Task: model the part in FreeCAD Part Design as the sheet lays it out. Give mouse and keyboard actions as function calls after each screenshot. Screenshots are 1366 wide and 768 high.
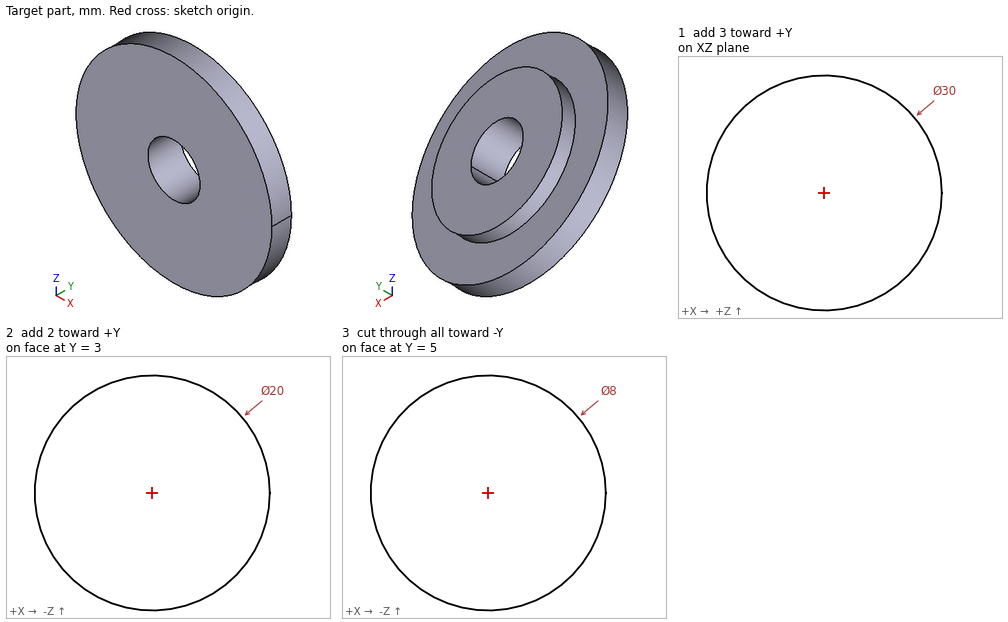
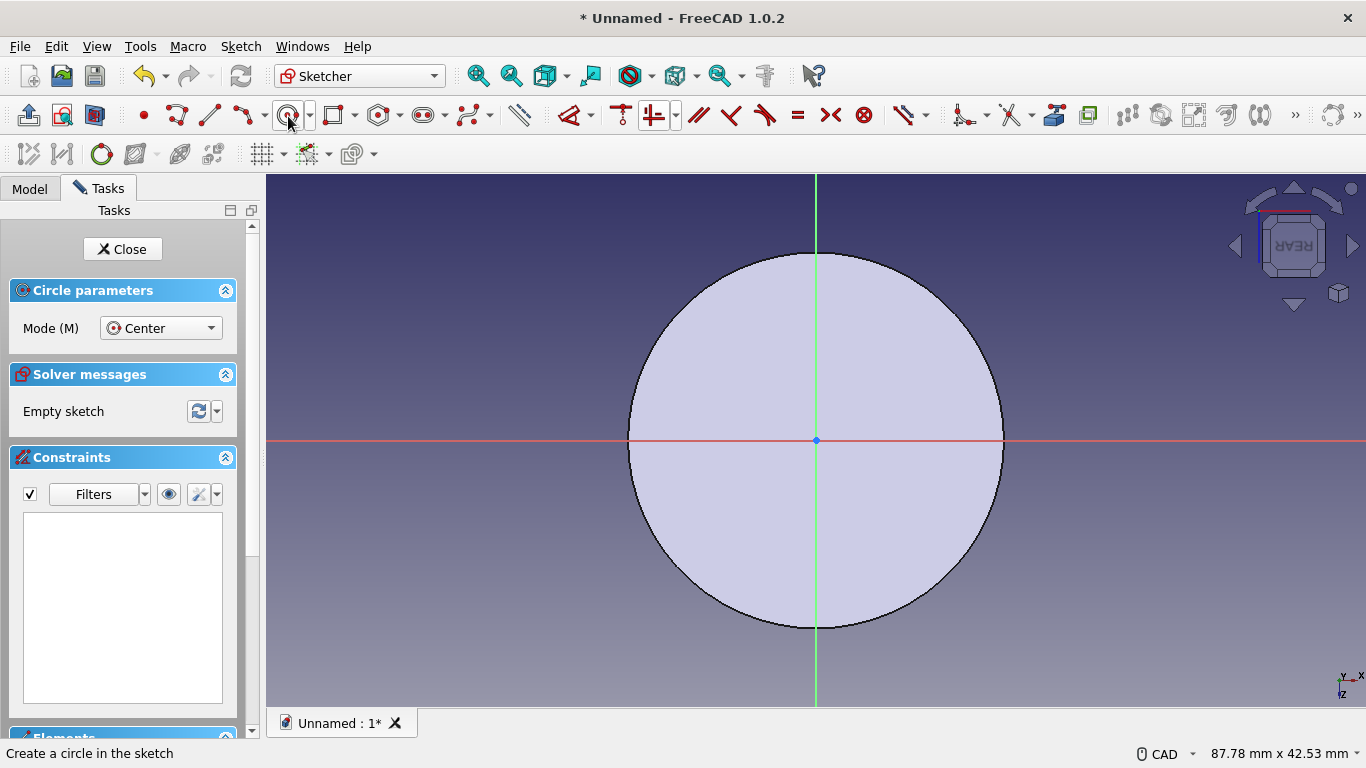
click(816, 441)
click(905, 352)
key(Escape)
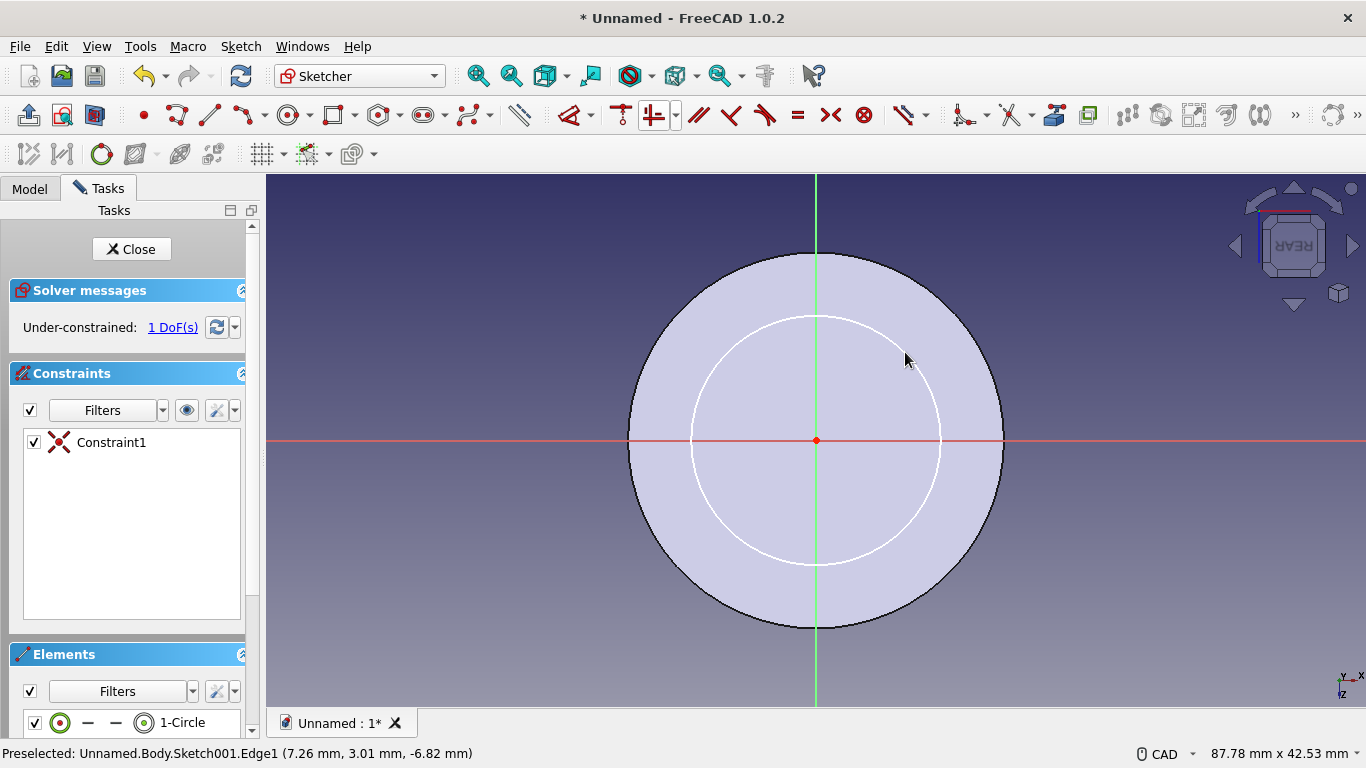
click(568, 116)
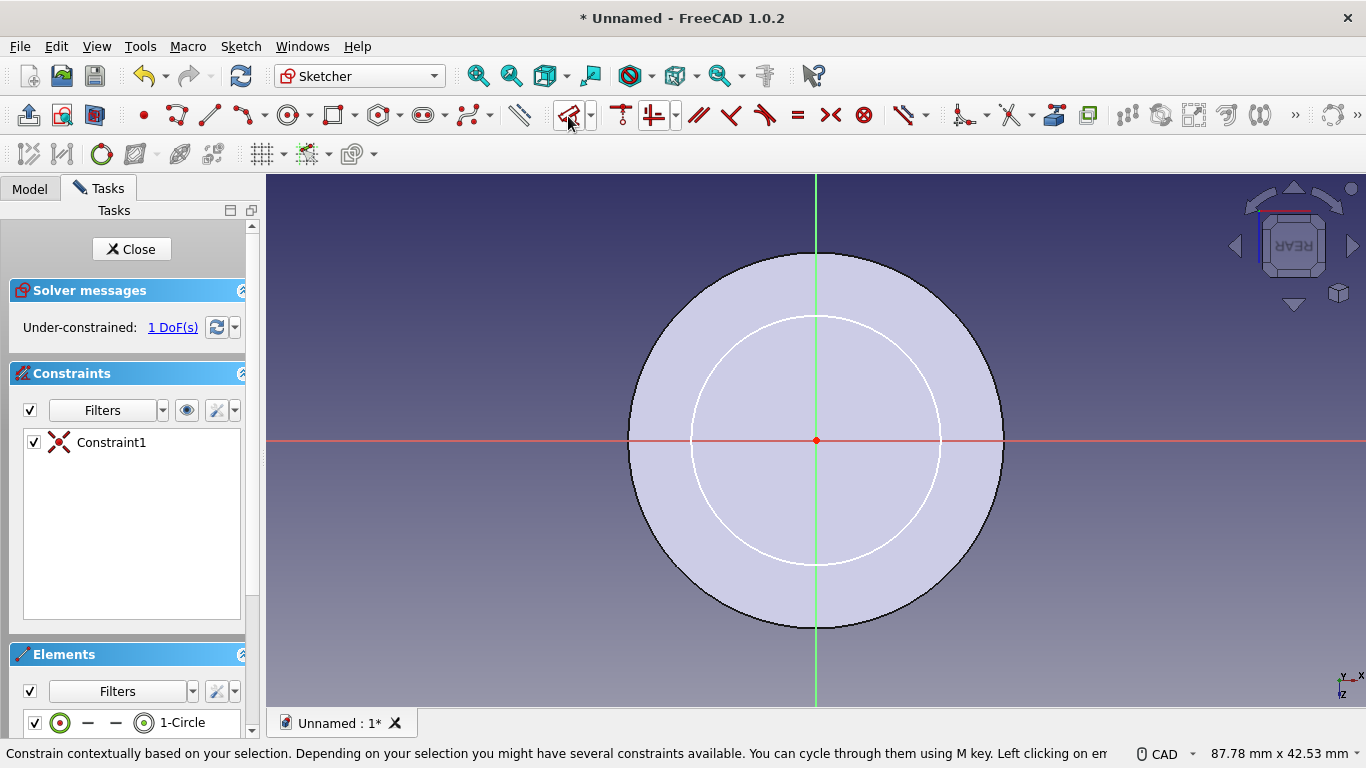
click(904, 352)
click(927, 329)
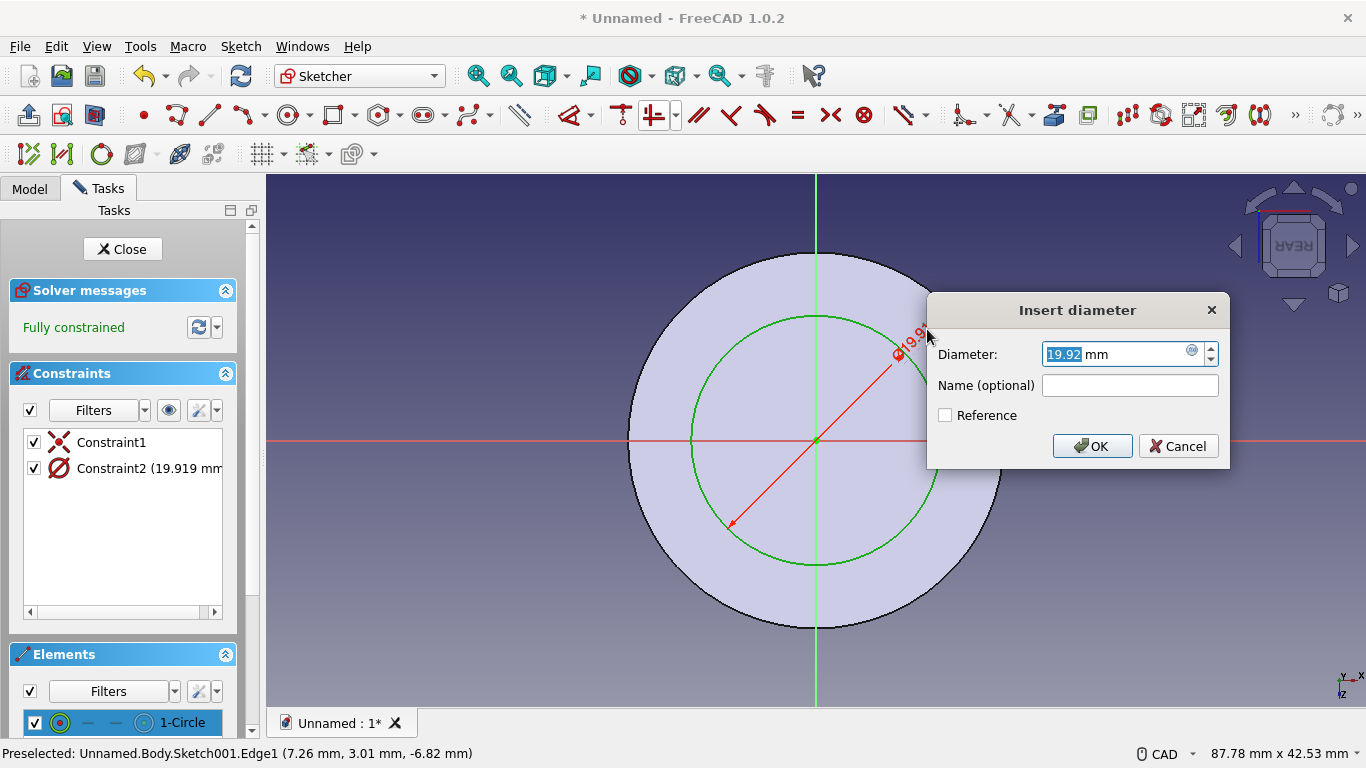
text(20)
key(Return)
key(Escape)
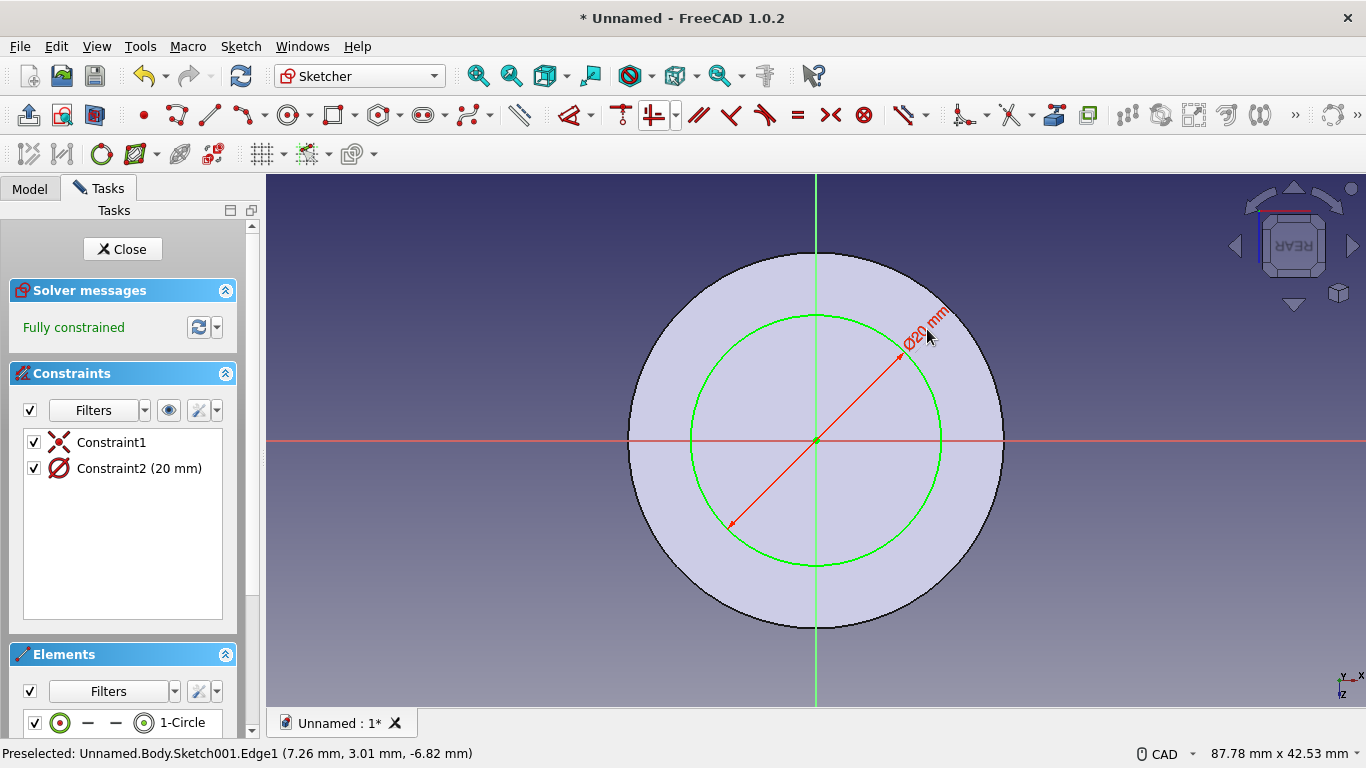
click(123, 249)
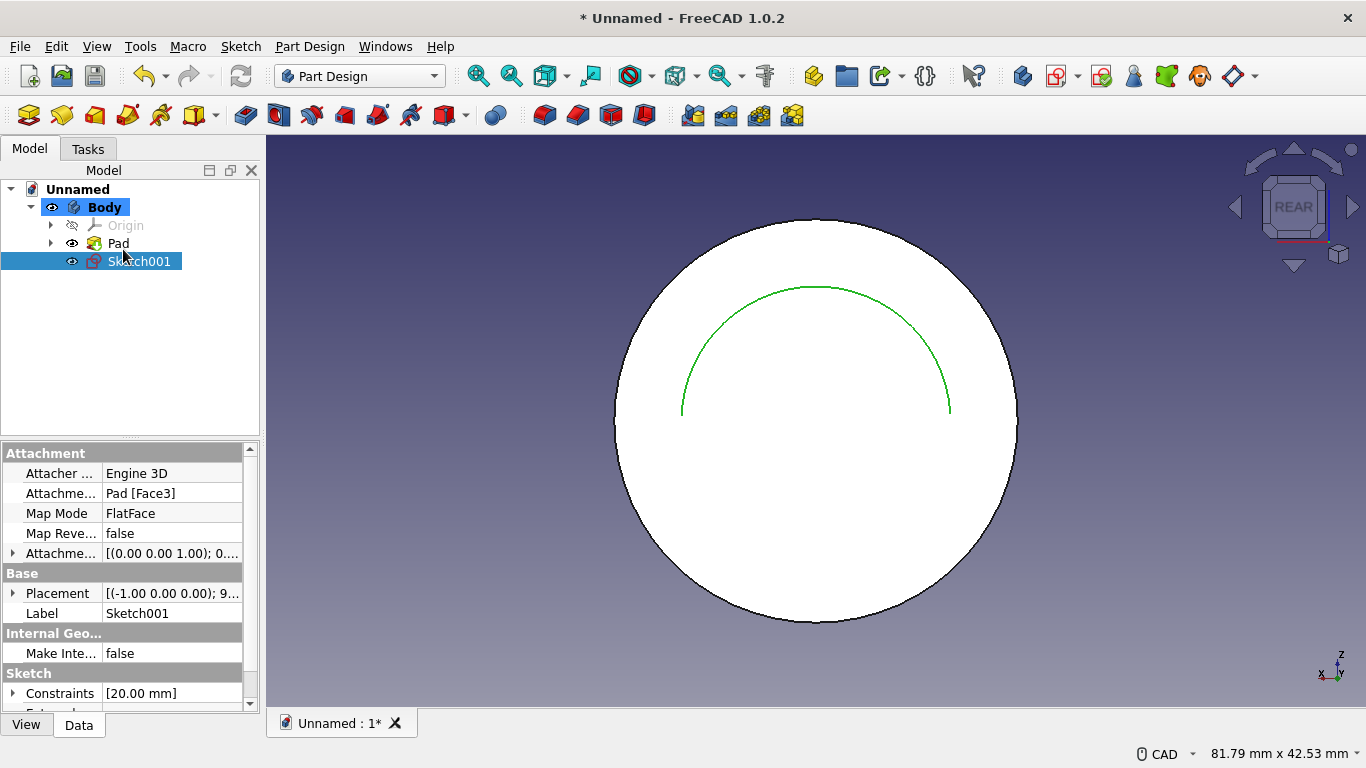
click(29, 116)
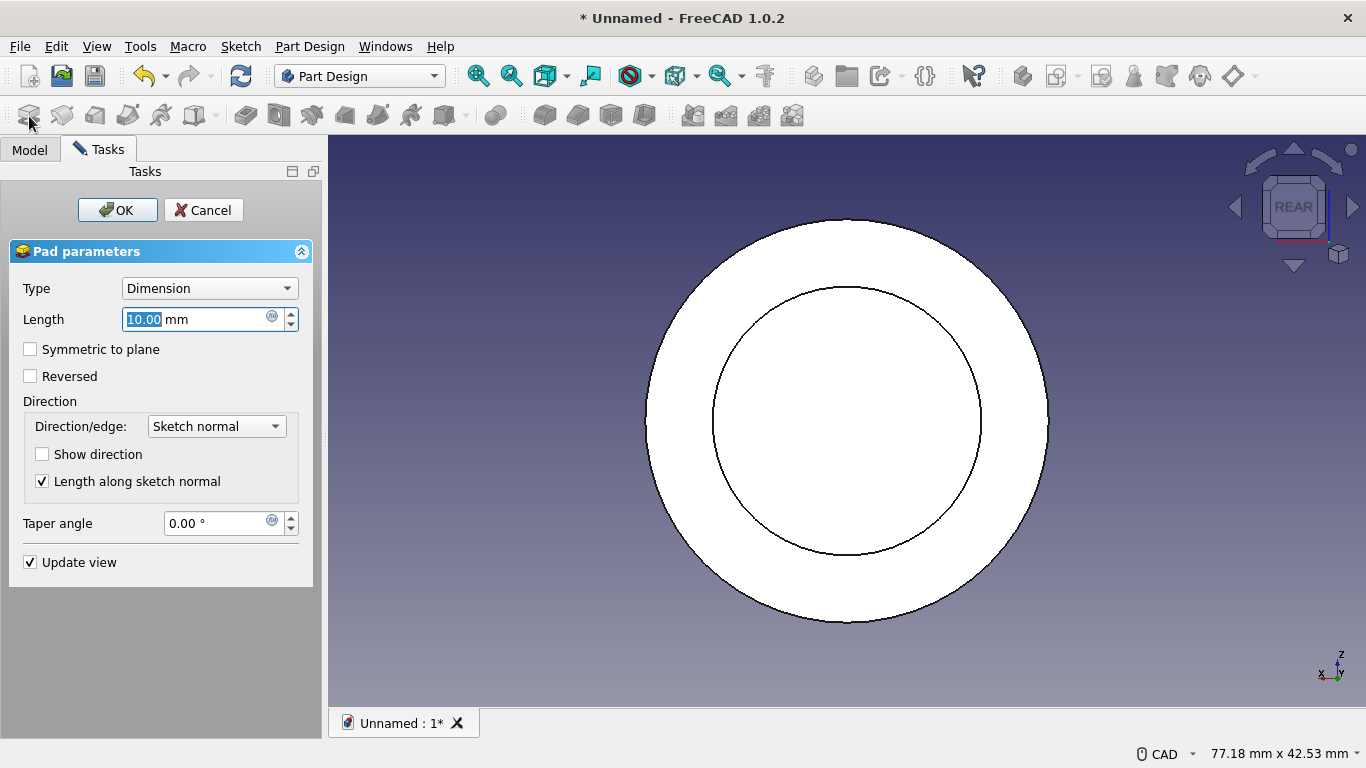
text(2)
key(Tab)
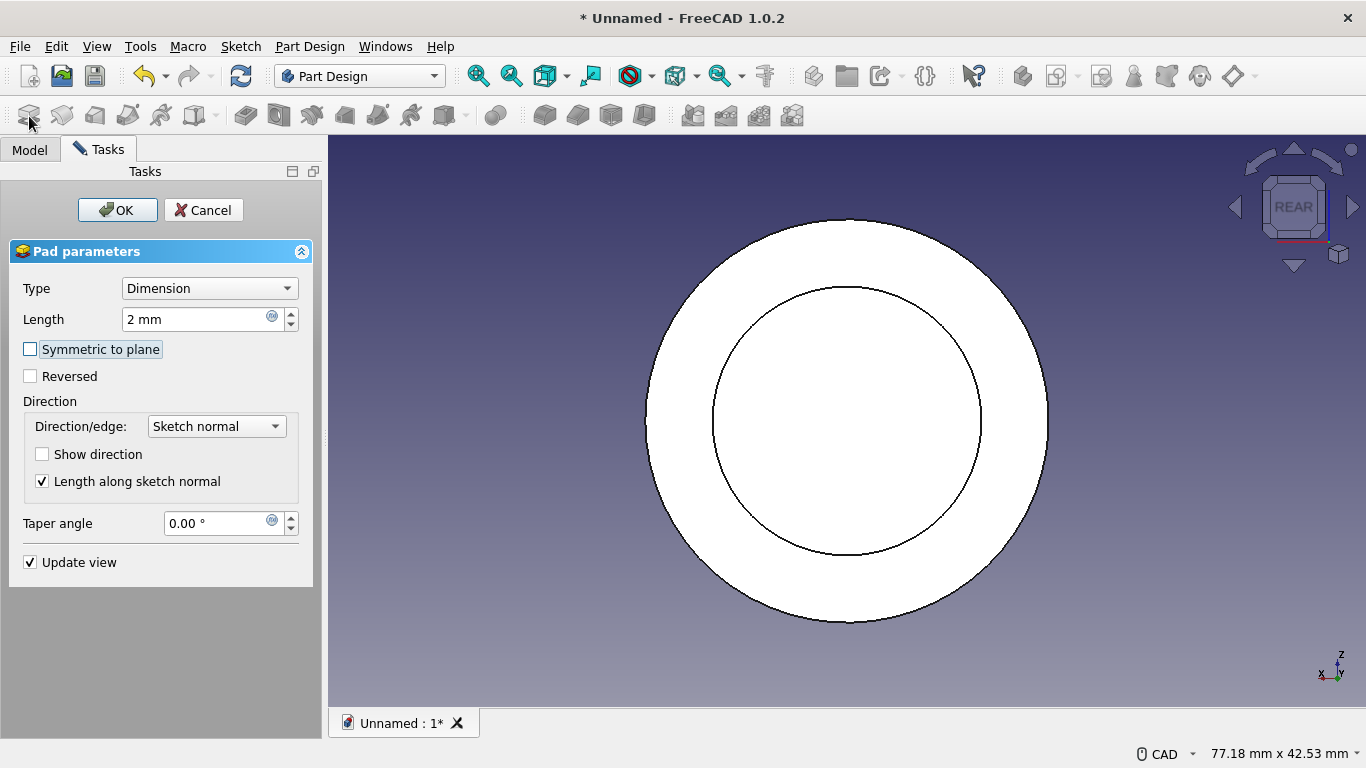
click(118, 210)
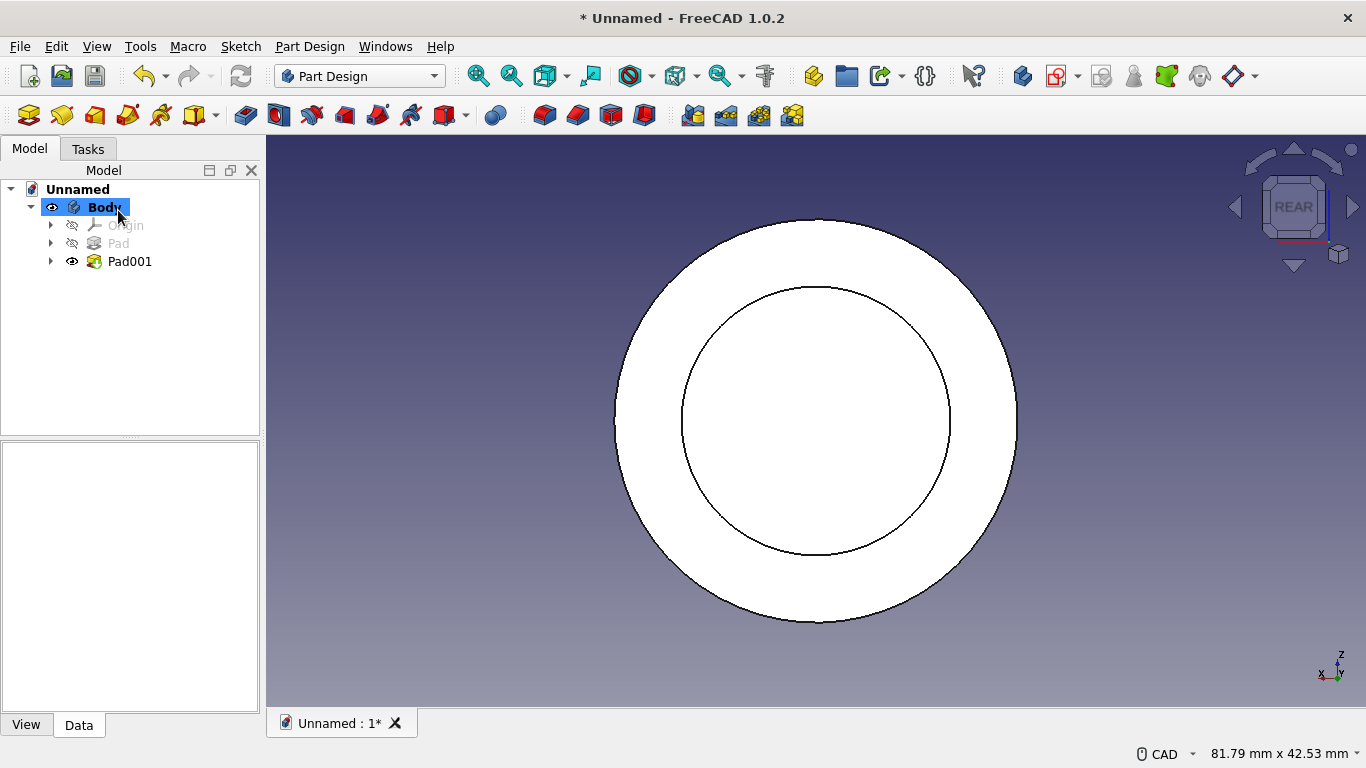
click(816, 420)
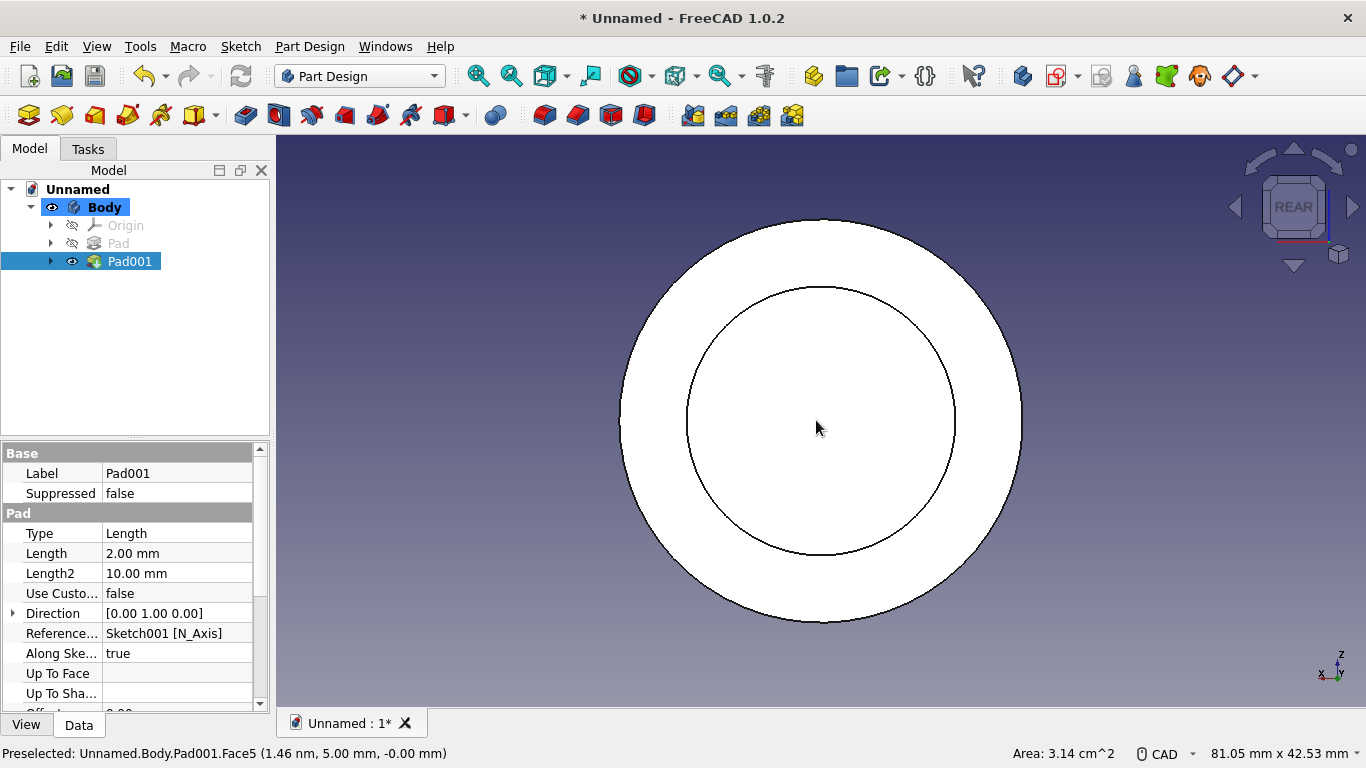
click(1056, 76)